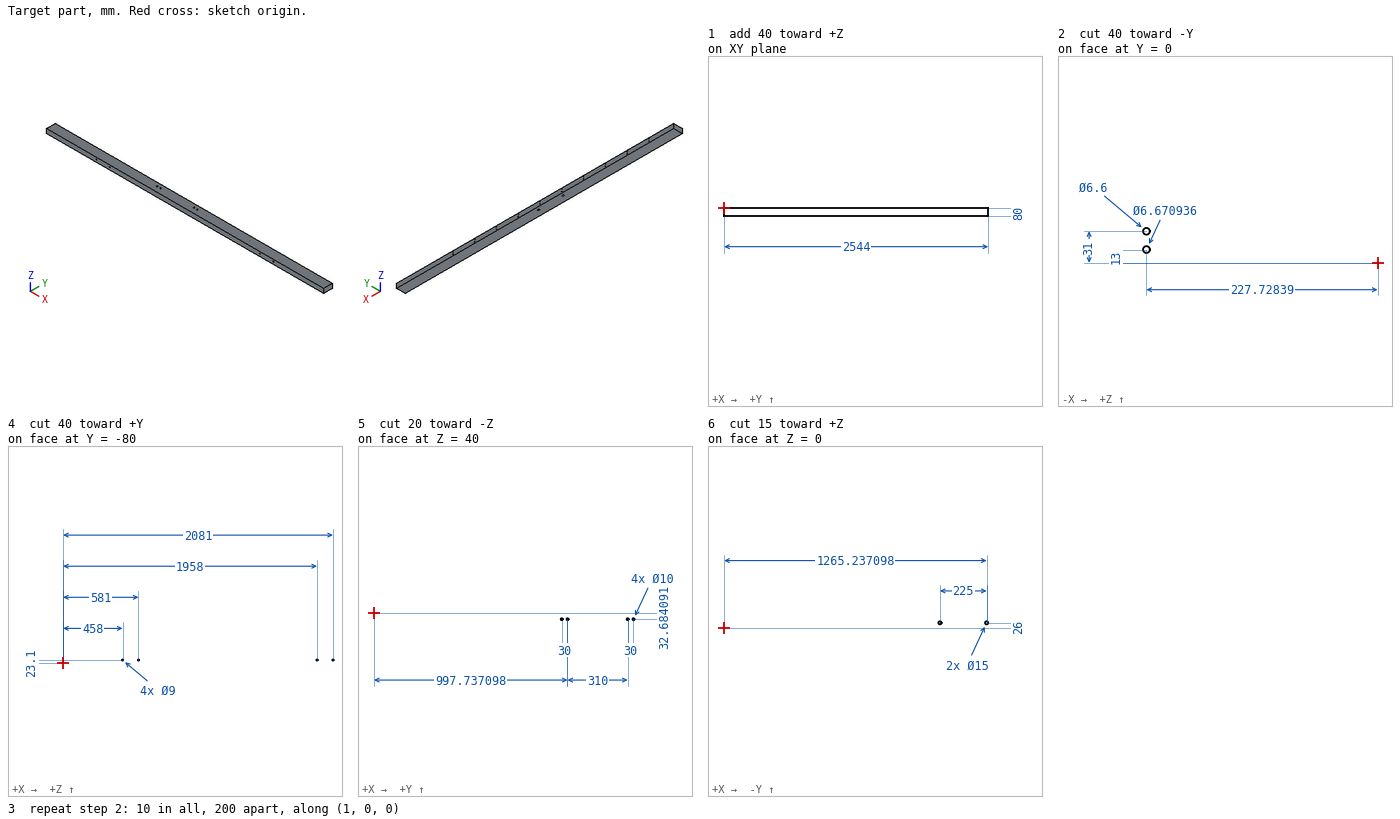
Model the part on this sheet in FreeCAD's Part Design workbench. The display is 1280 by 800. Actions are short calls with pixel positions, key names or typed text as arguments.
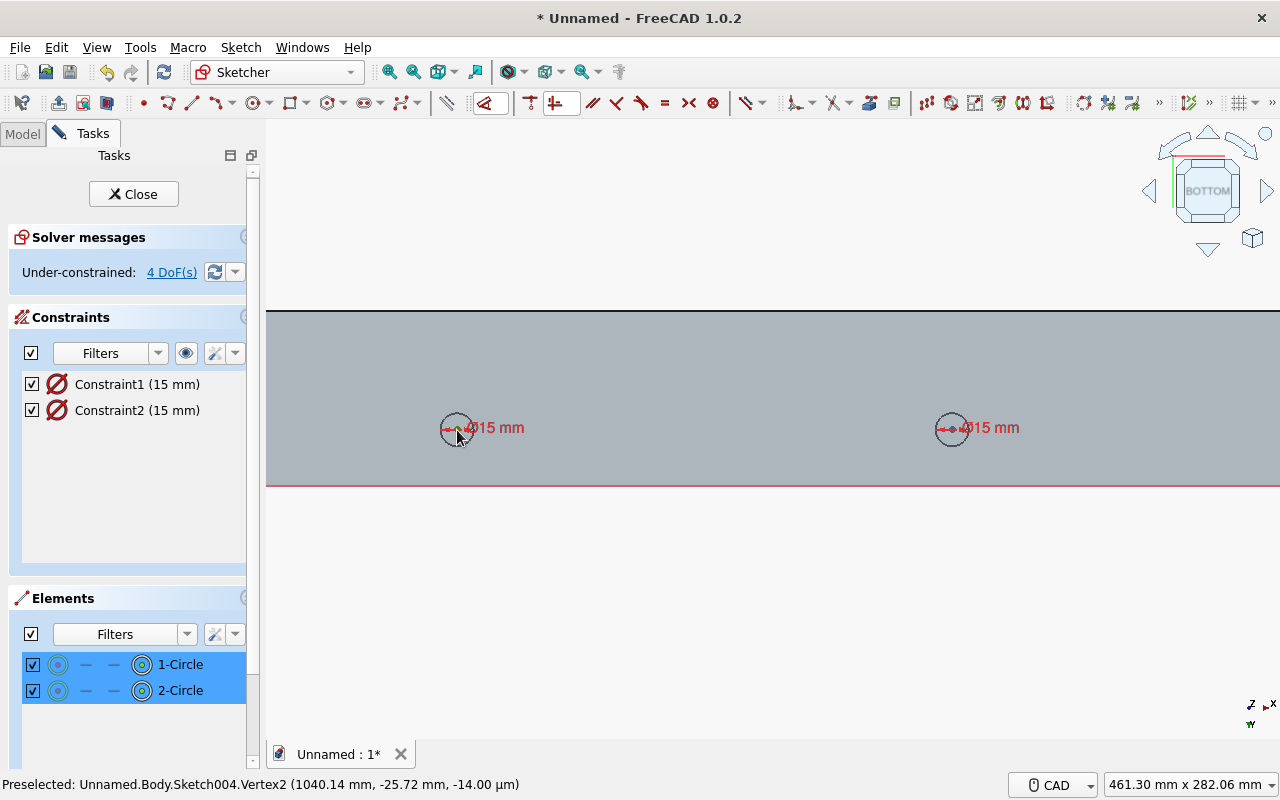
key(h)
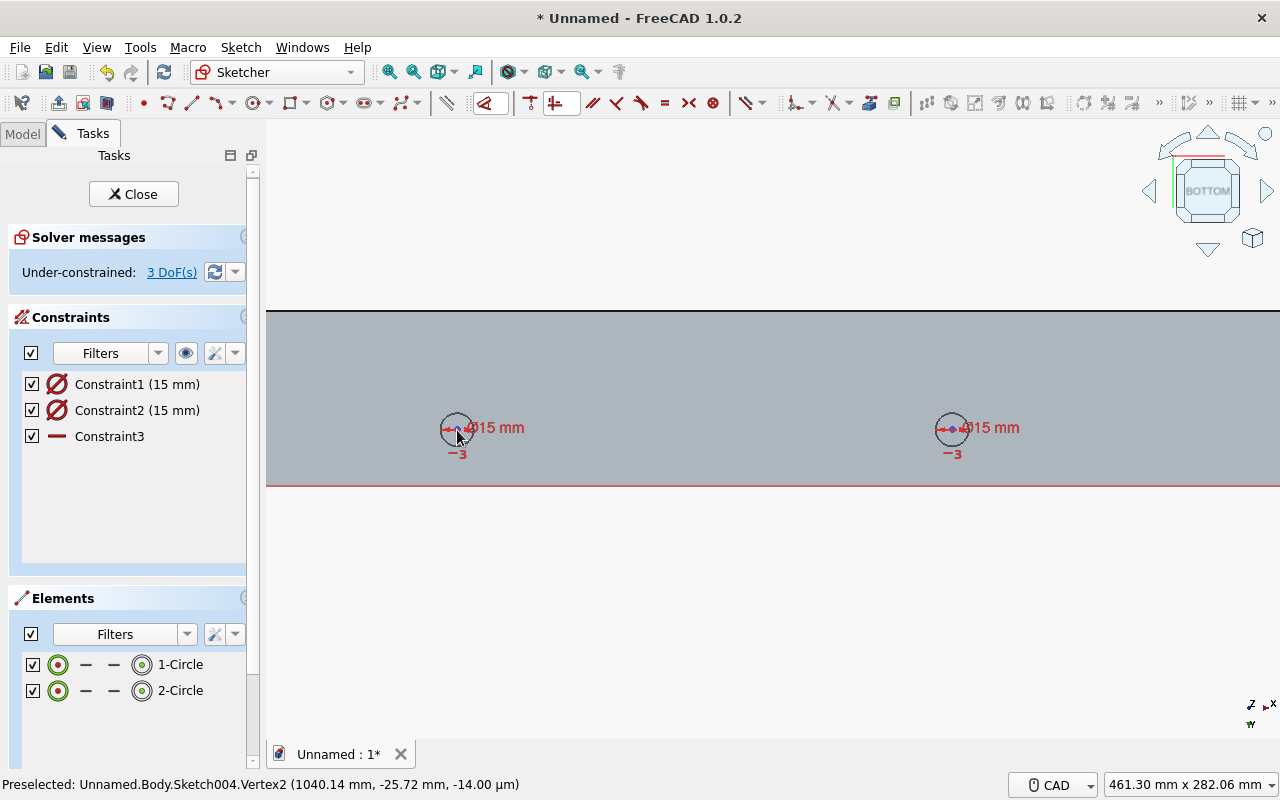
key(d)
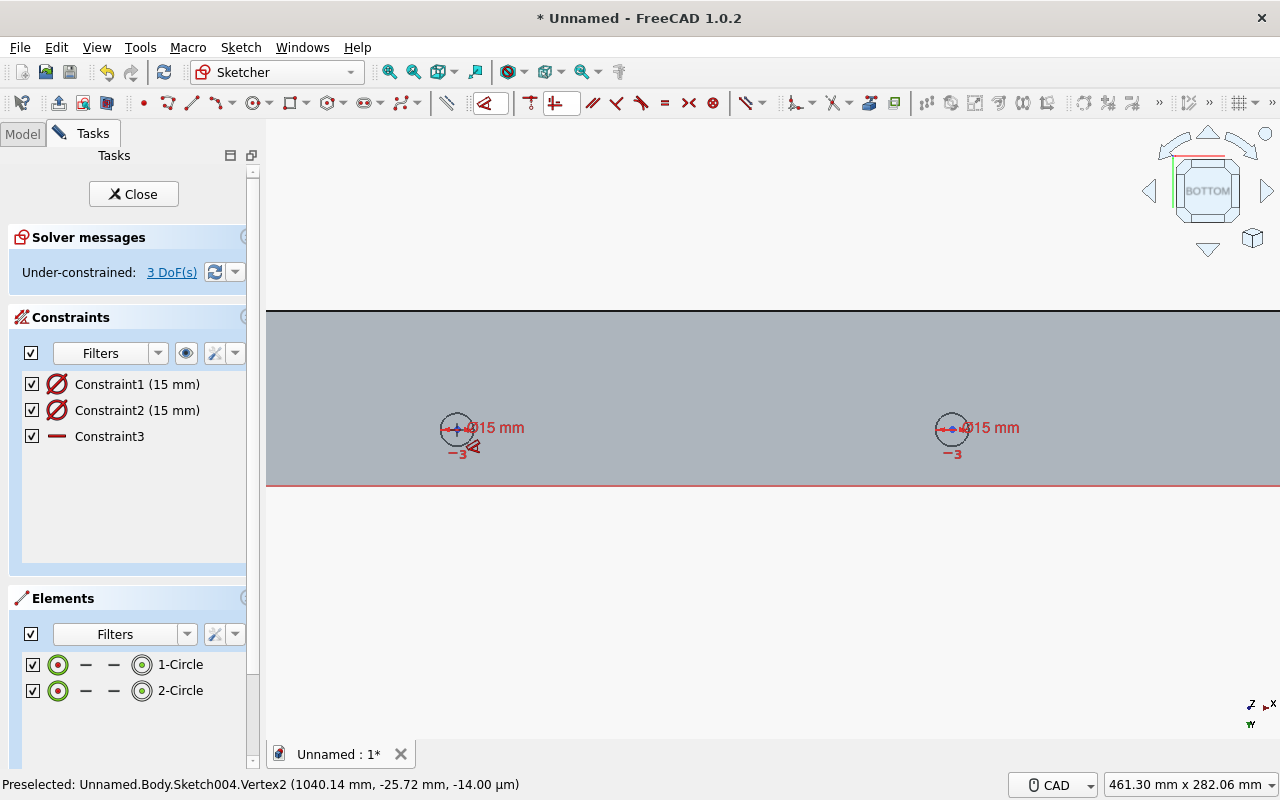
click(952, 430)
click(986, 458)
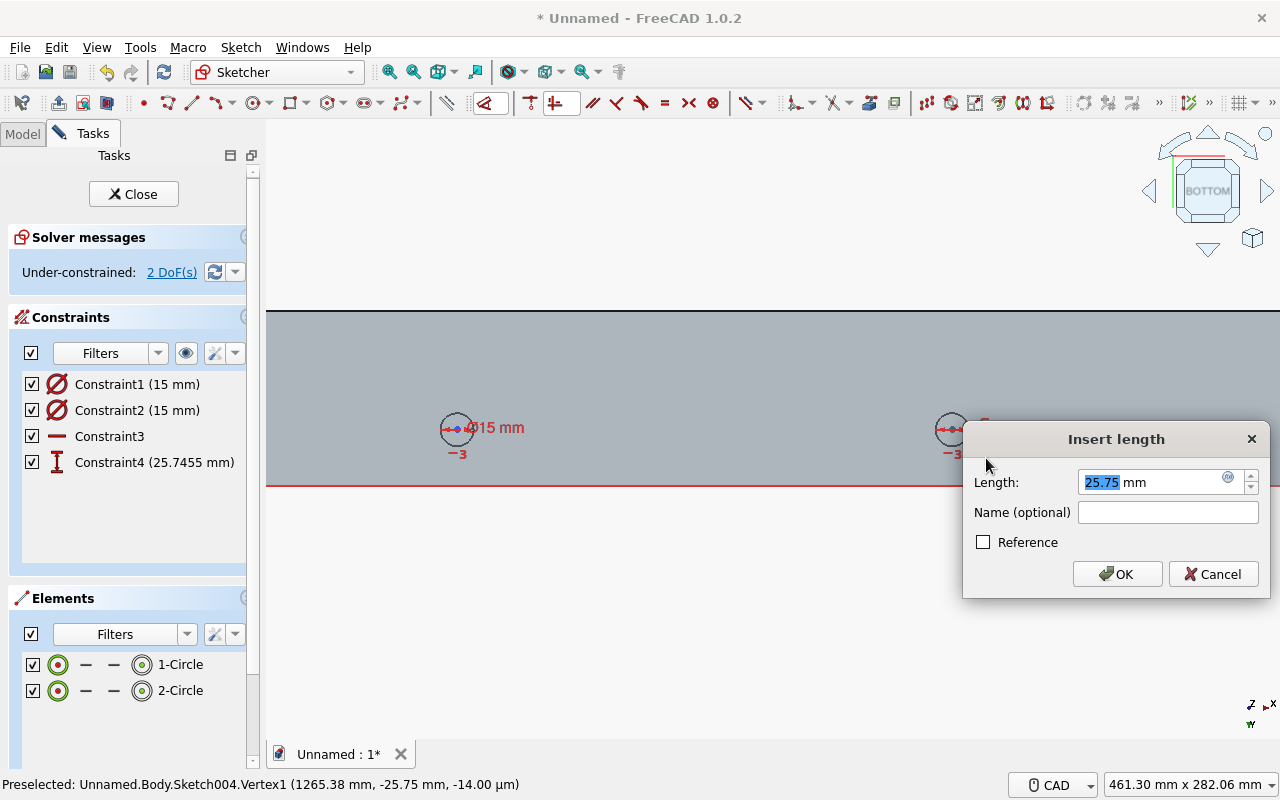
text(26)
key(Return)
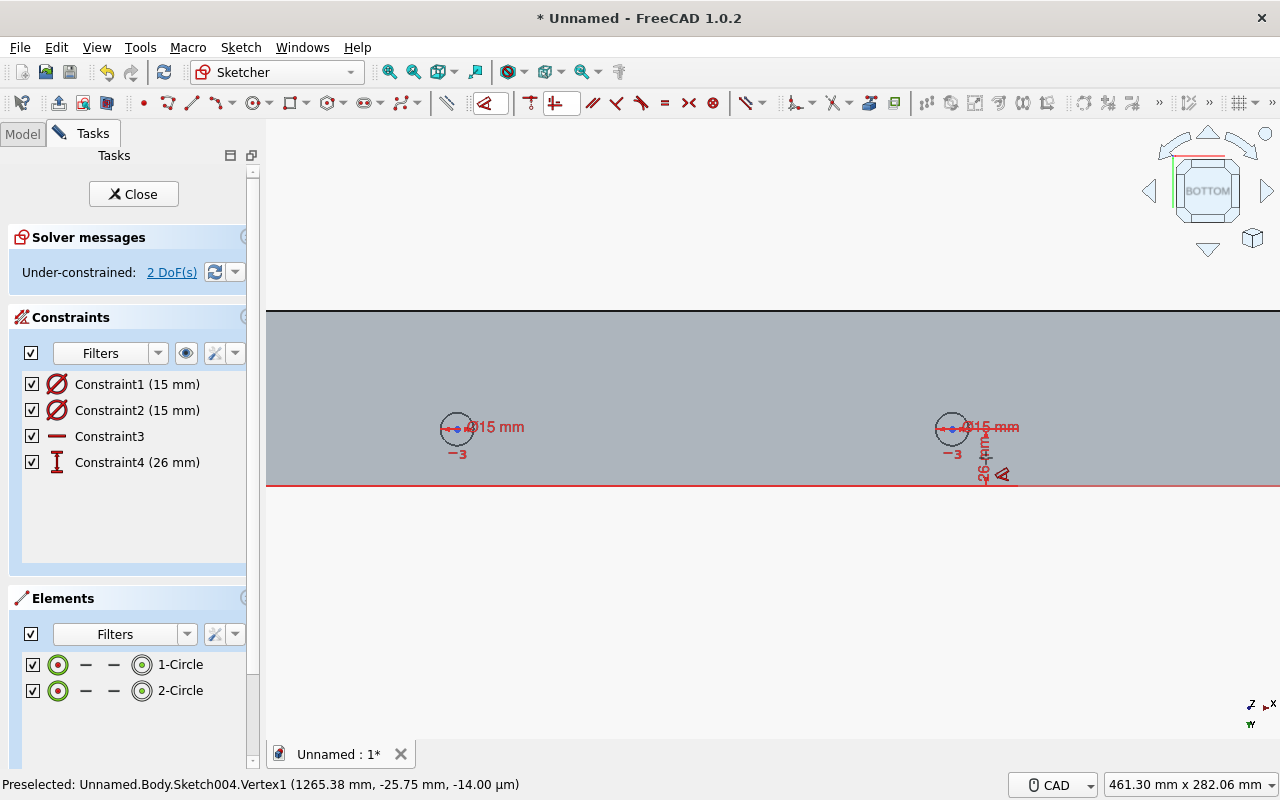
click(952, 429)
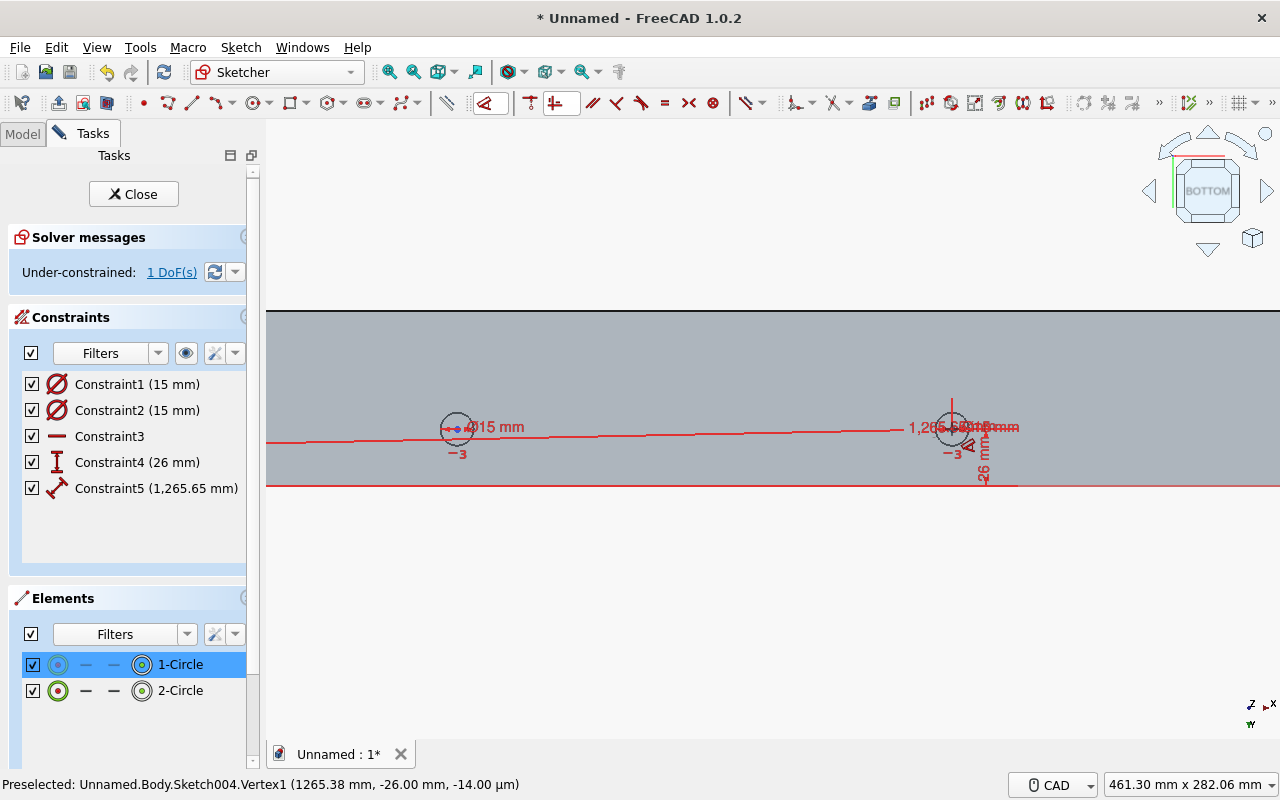
click(457, 429)
click(705, 463)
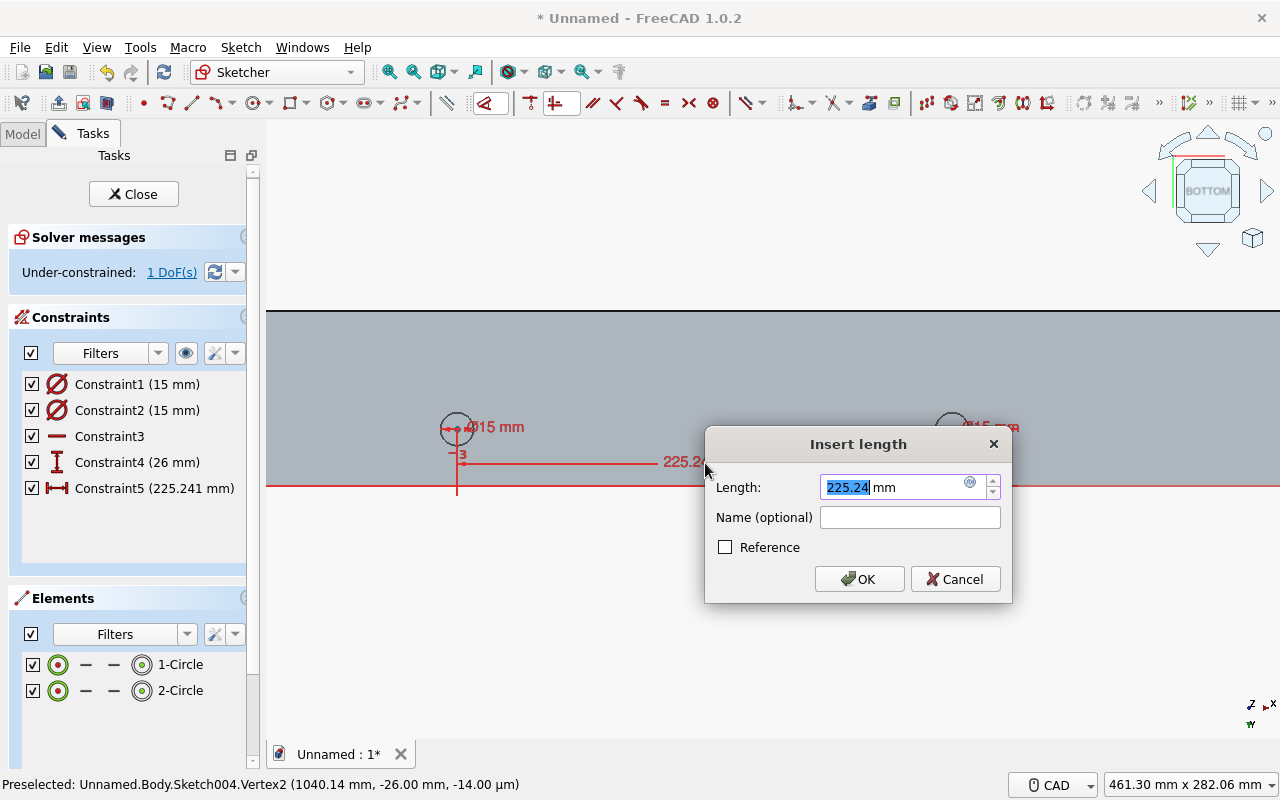
text(225)
key(Return)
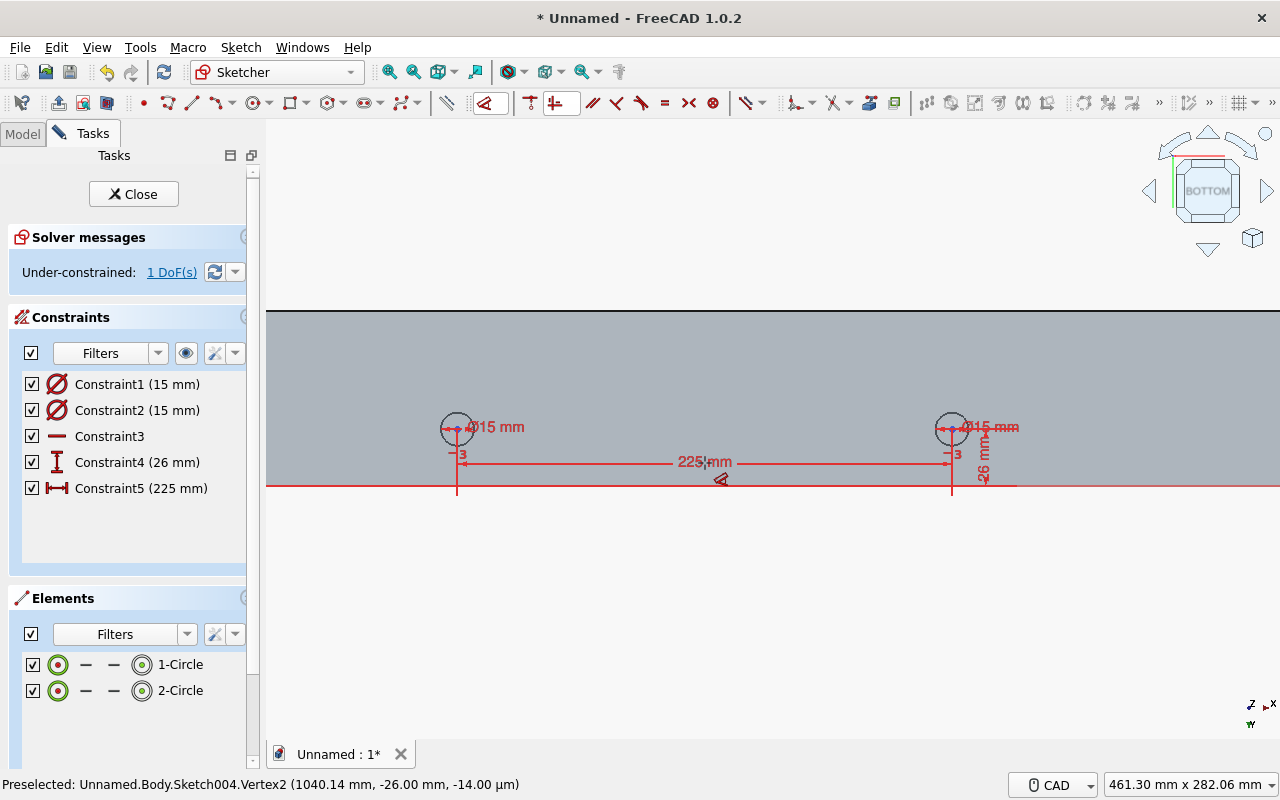
click(952, 429)
click(623, 520)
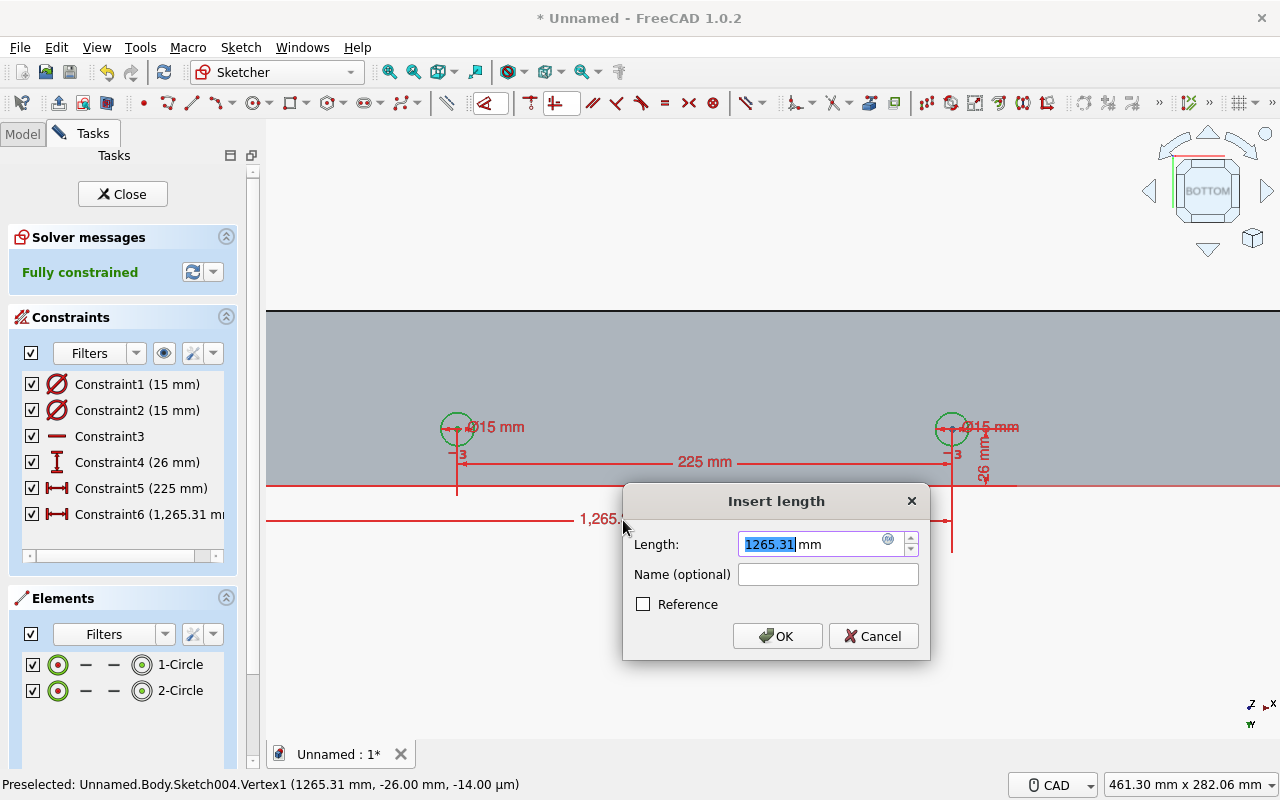
text(1265.237098)
key(Return)
key(Escape)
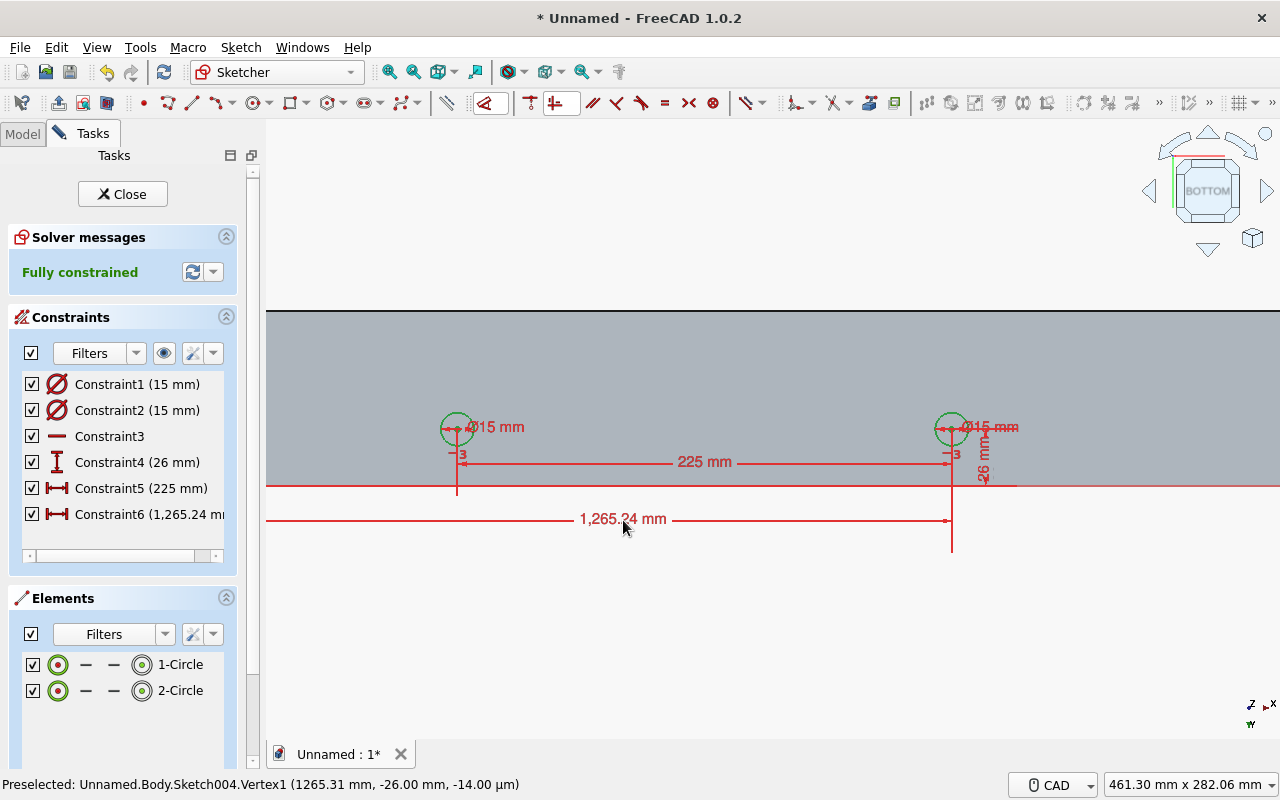
click(123, 194)